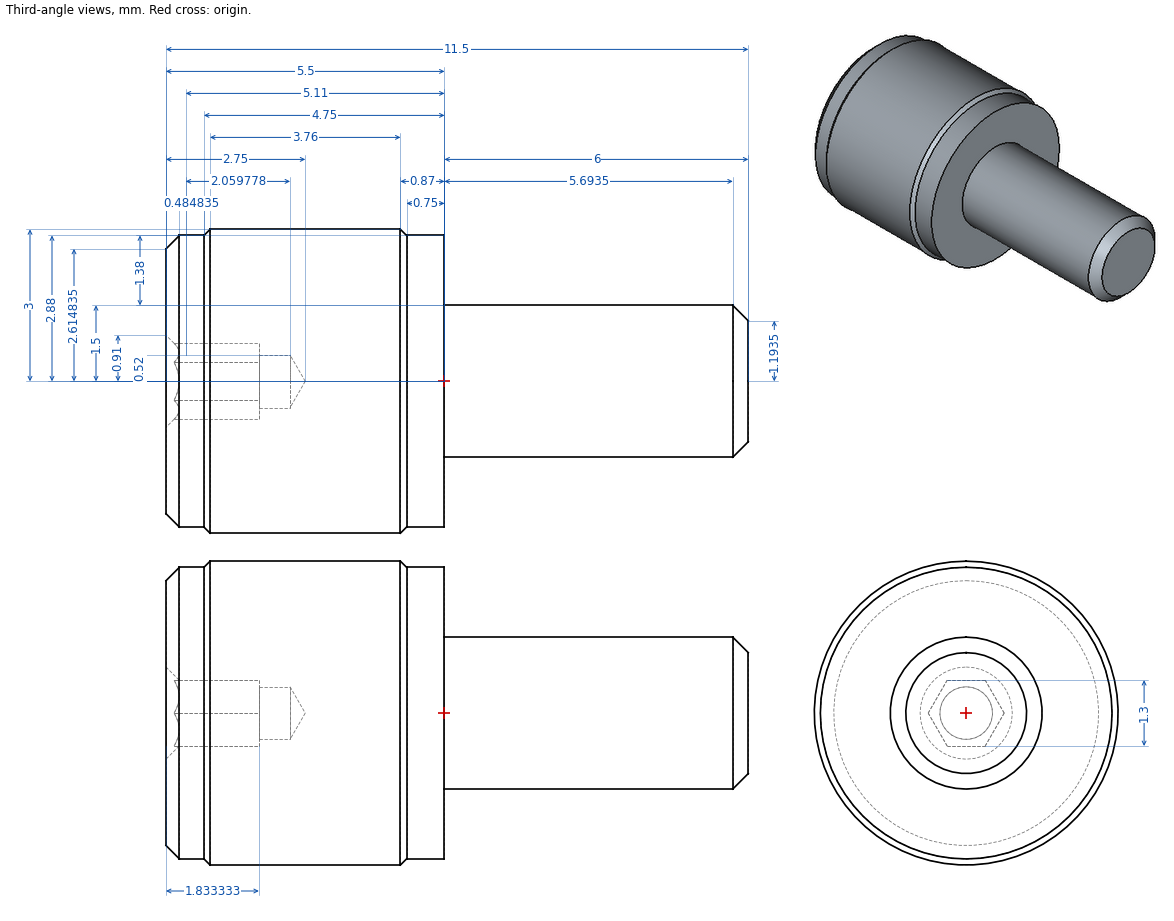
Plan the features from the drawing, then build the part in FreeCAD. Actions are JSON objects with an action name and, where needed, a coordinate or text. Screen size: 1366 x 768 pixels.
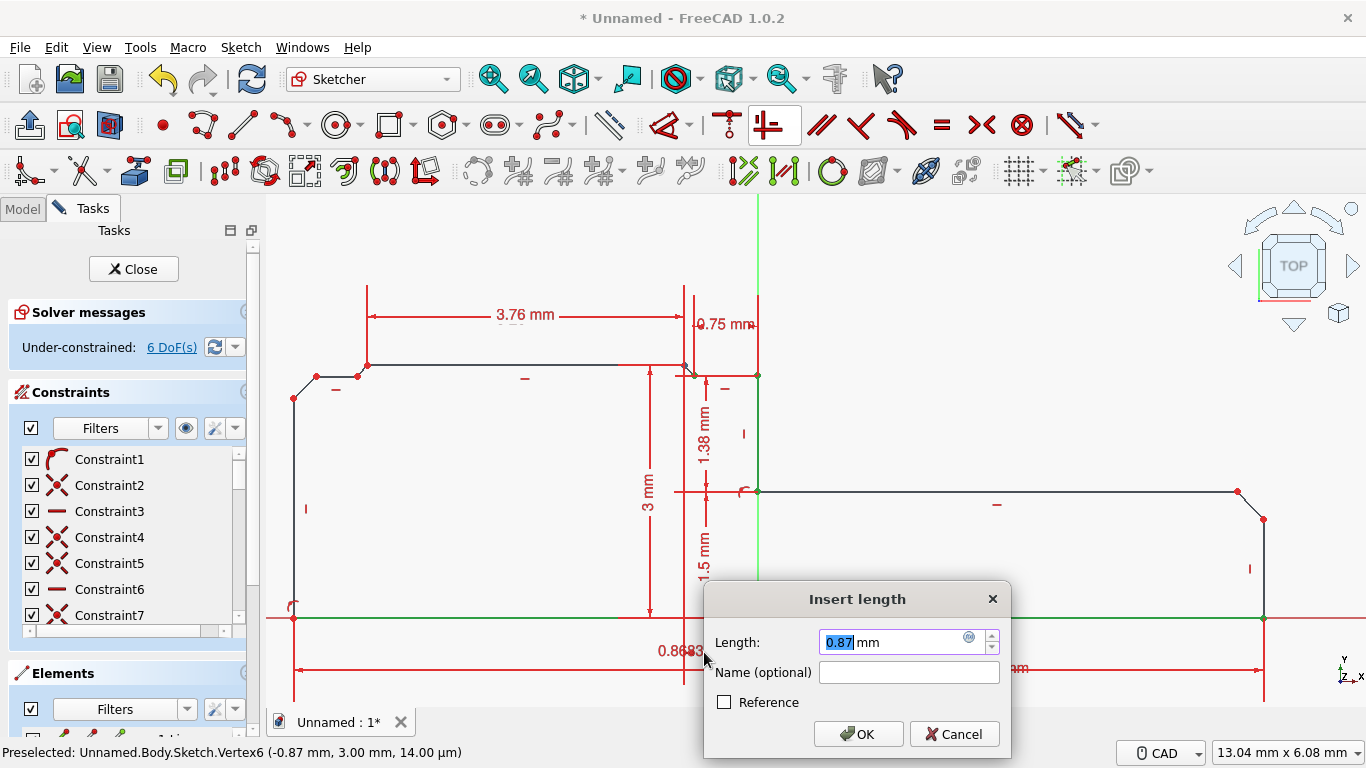
{"action": "type", "text": "0.87"}
{"action": "key", "text": "Return"}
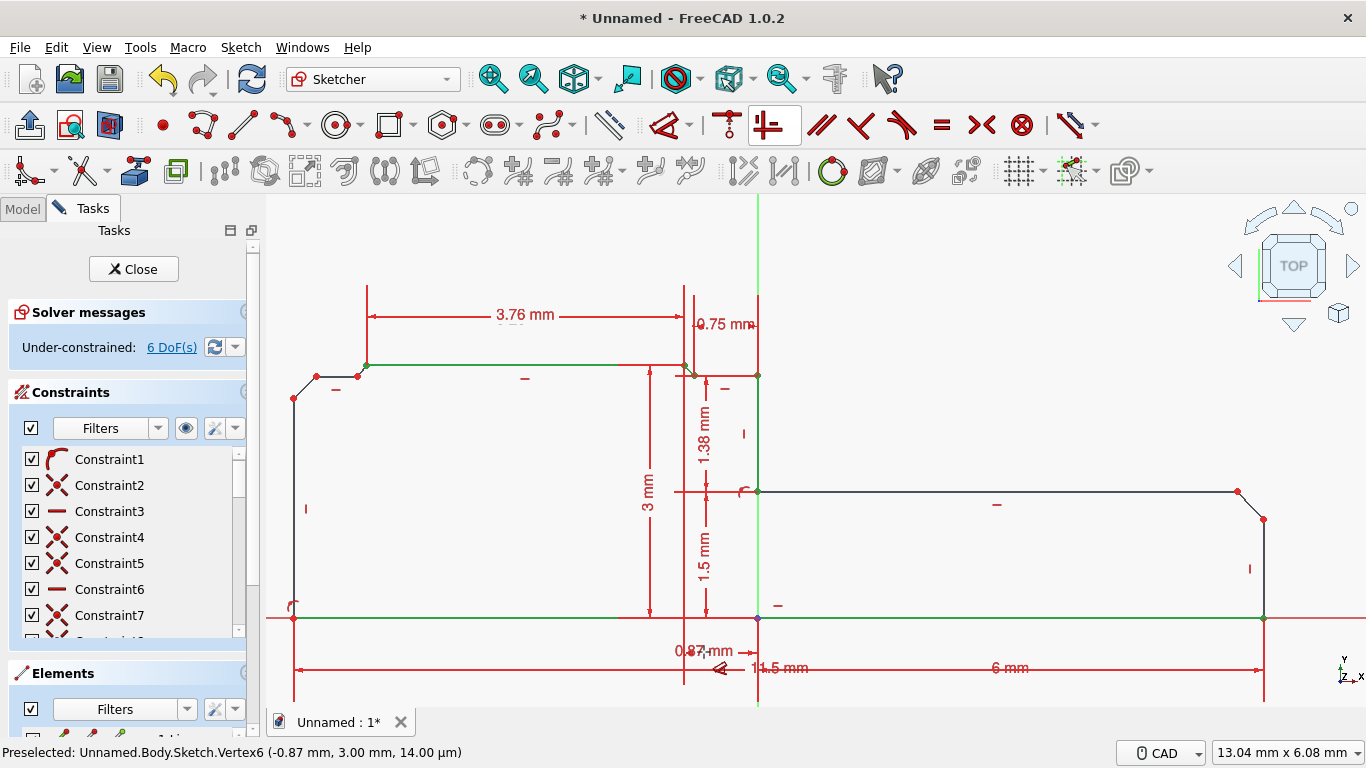
{"action": "left_click", "coordinate": [357, 377]}
{"action": "left_click", "coordinate": [557, 652]}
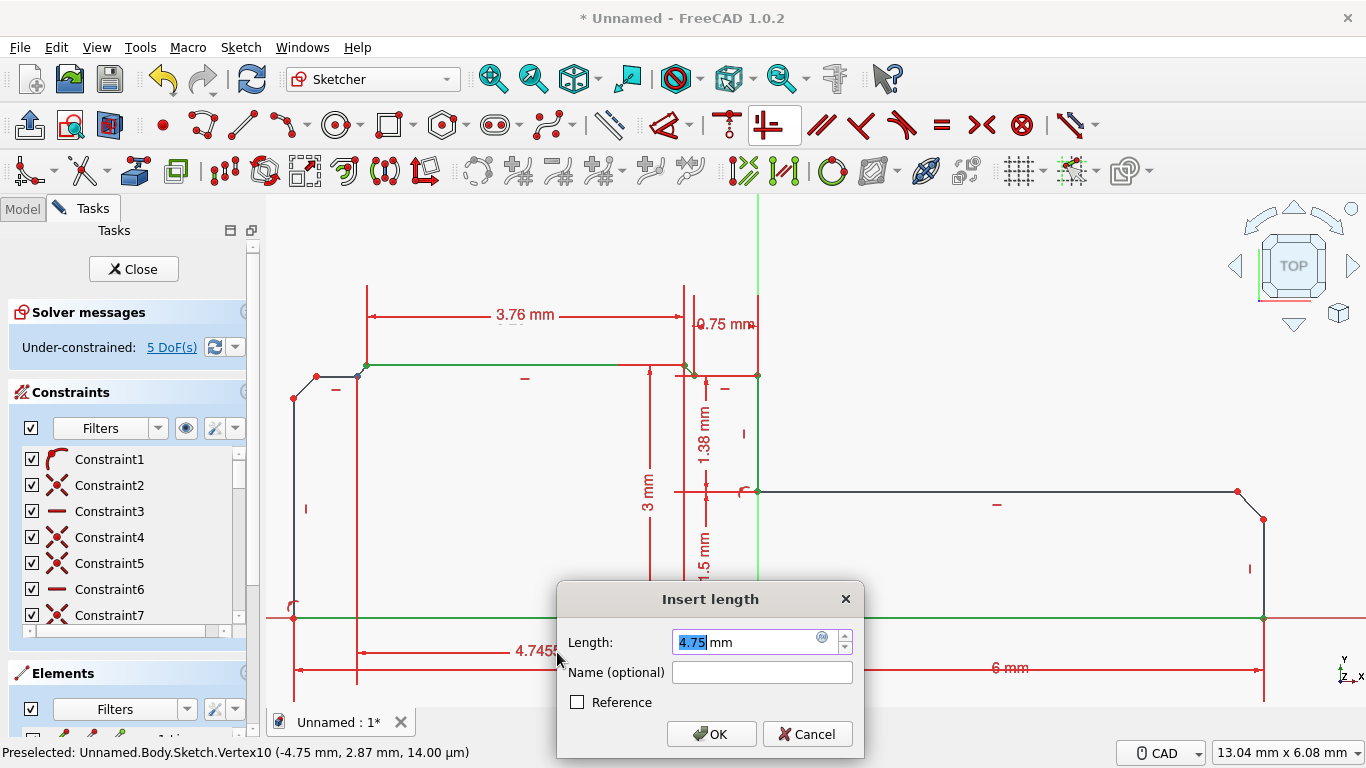
{"action": "type", "text": "4.75"}
{"action": "key", "text": "Return"}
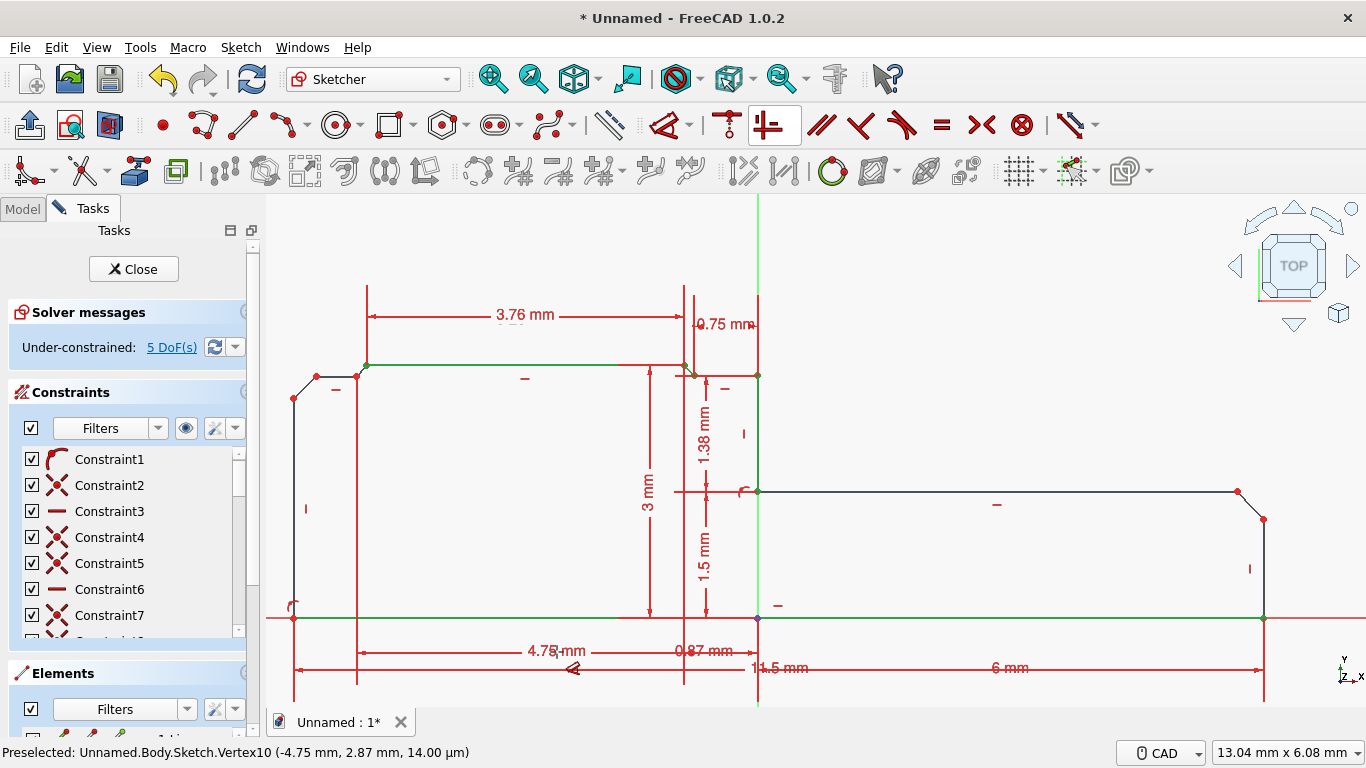
{"action": "left_click", "coordinate": [357, 377]}
{"action": "left_click", "coordinate": [323, 498]}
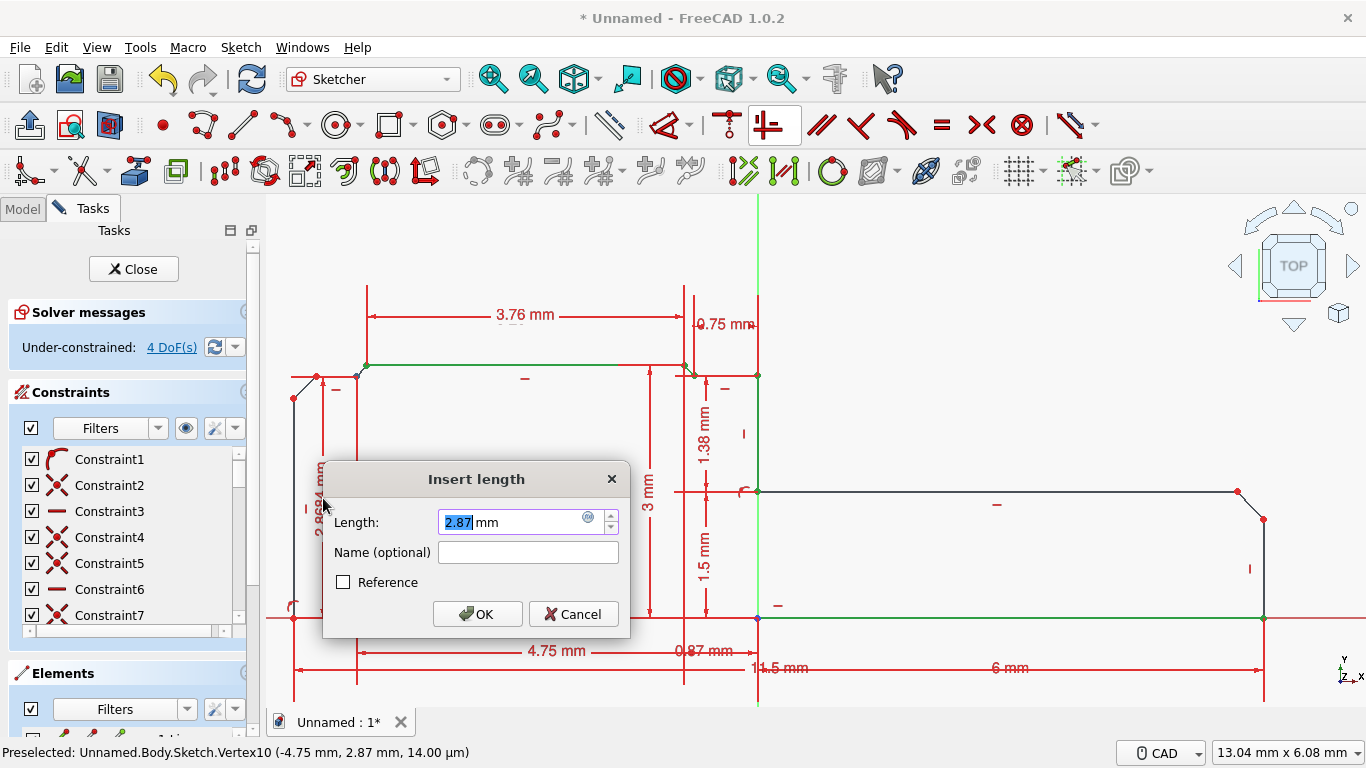
{"action": "type", "text": "2.88"}
{"action": "key", "text": "Return"}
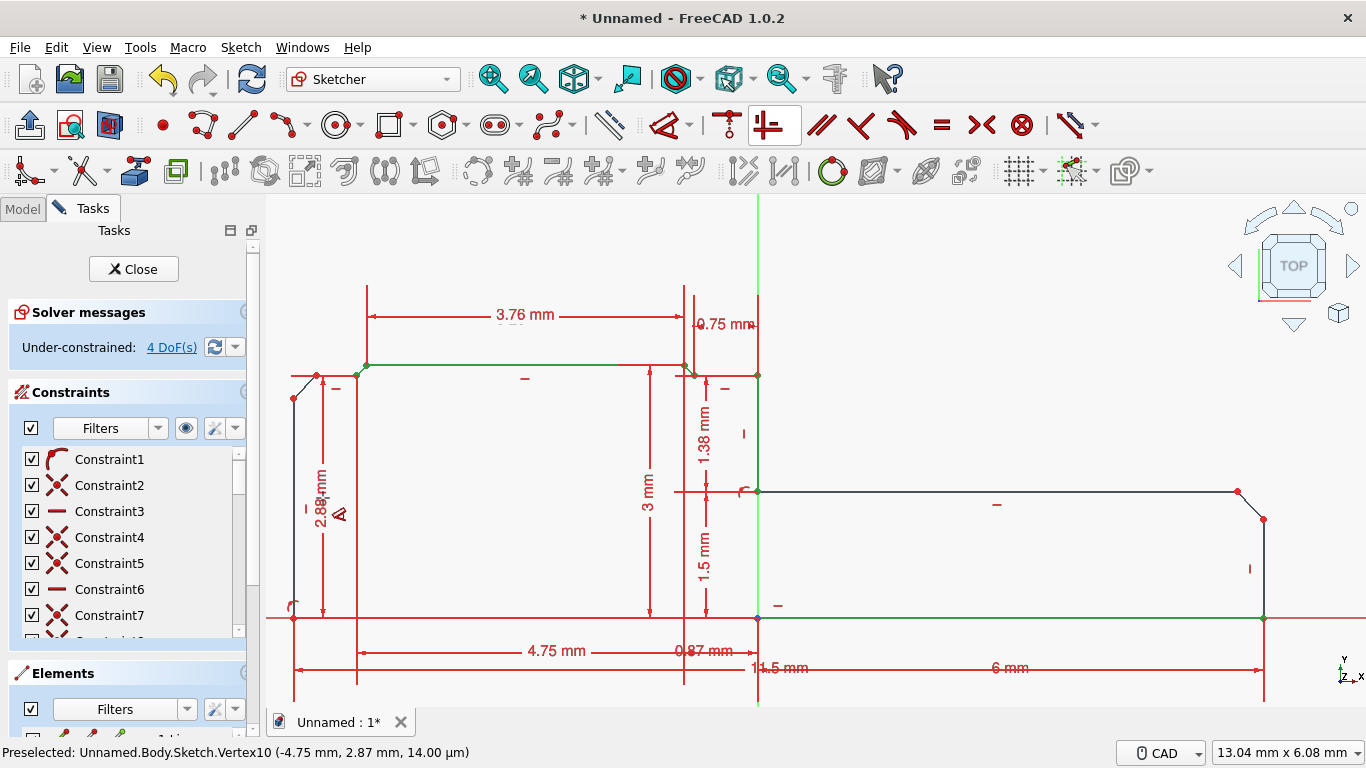
{"action": "scroll", "coordinate": [684, 366], "scroll_direction": "down", "scroll_amount": 2}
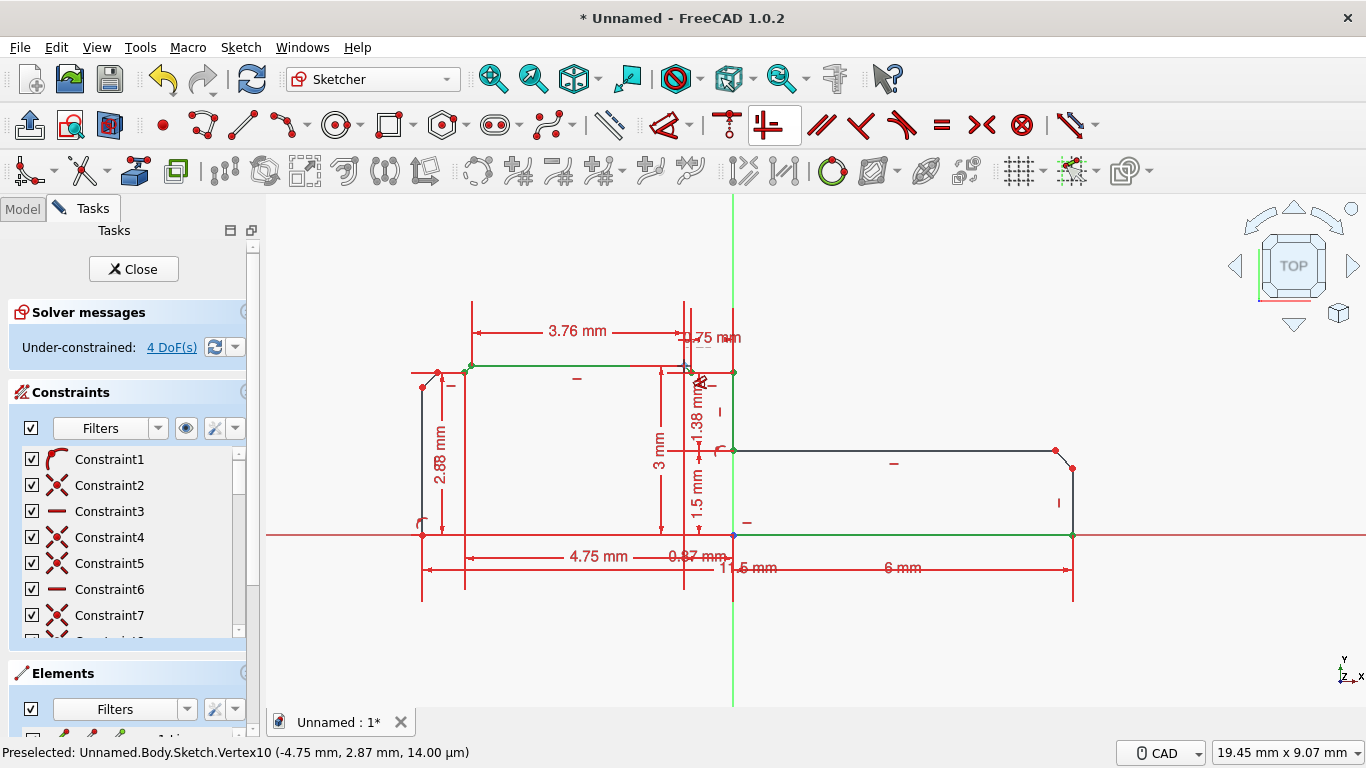
{"action": "left_click", "coordinate": [1073, 515]}
{"action": "left_click", "coordinate": [1107, 502]}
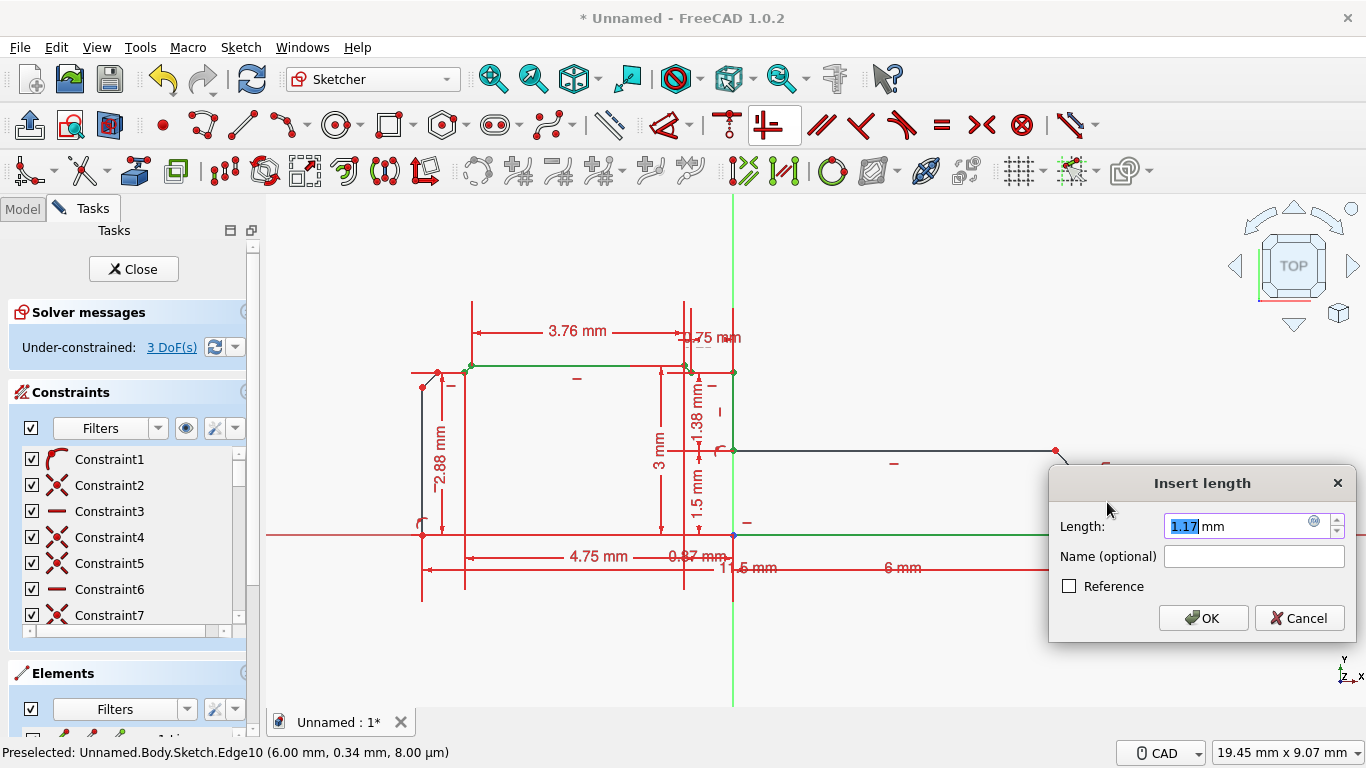
{"action": "type", "text": "1.1935"}
{"action": "key", "text": "Return"}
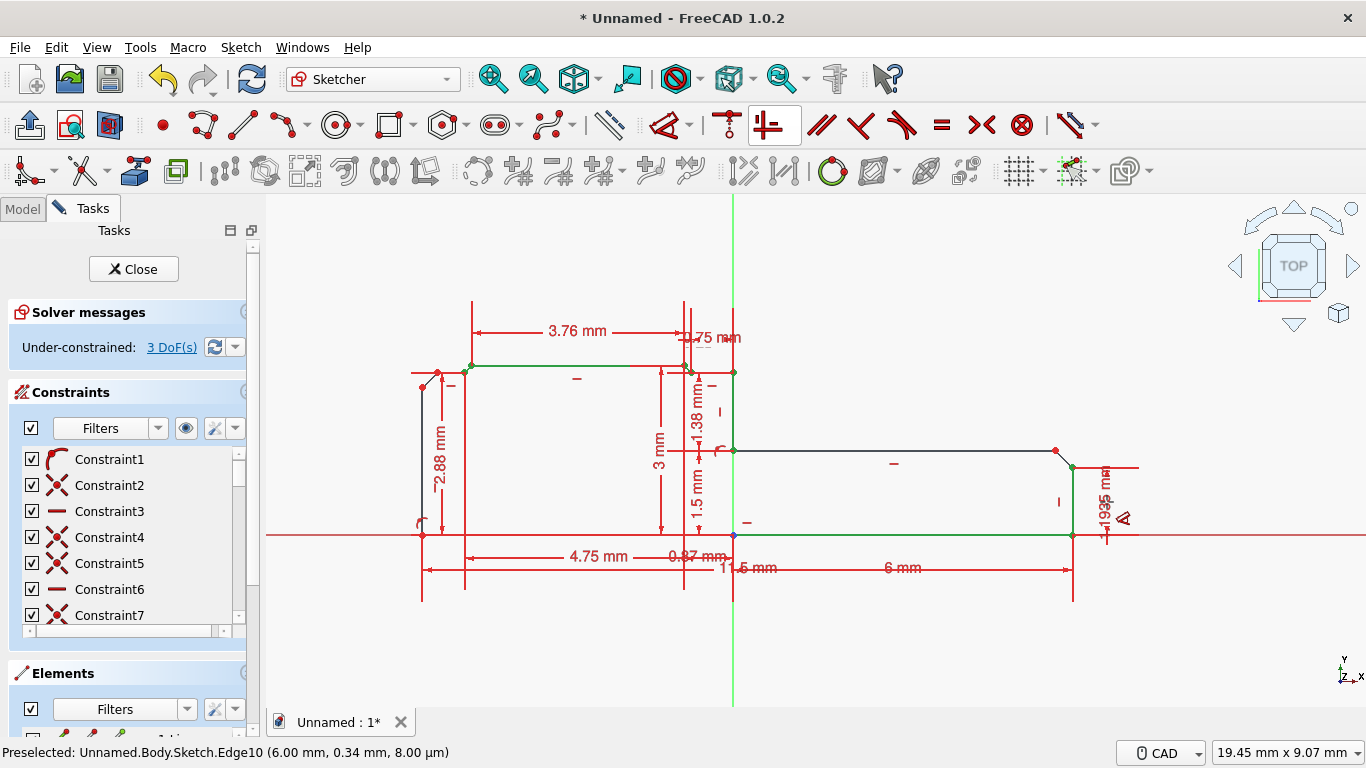
{"action": "left_click", "coordinate": [959, 451]}
{"action": "left_click", "coordinate": [894, 485]}